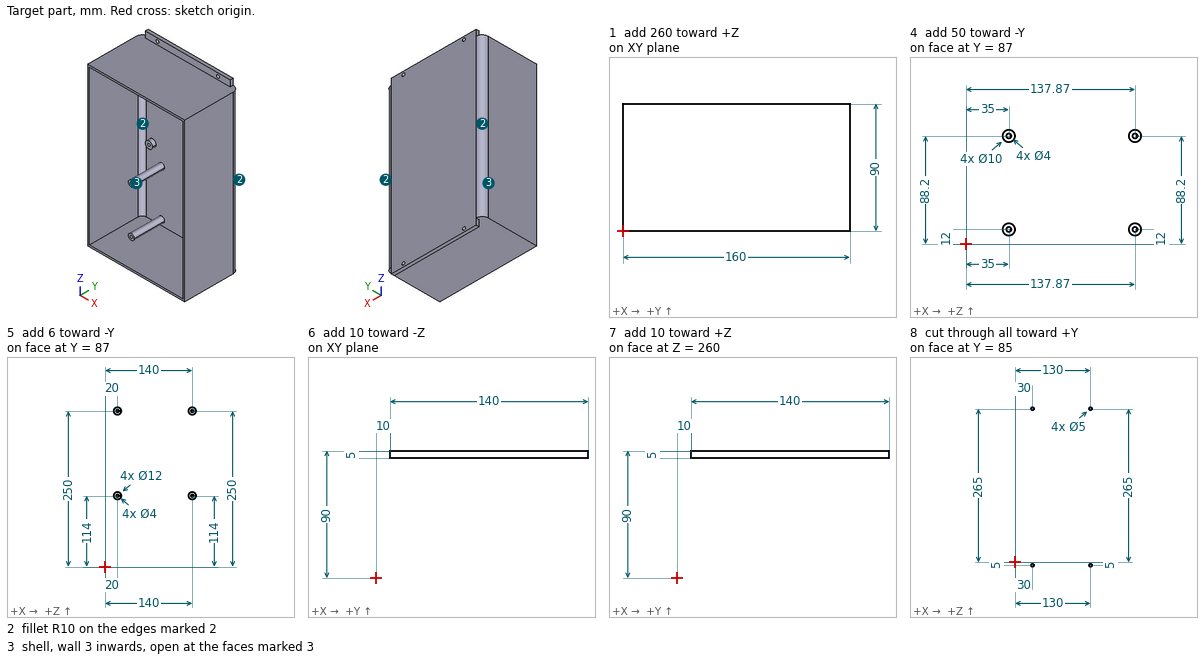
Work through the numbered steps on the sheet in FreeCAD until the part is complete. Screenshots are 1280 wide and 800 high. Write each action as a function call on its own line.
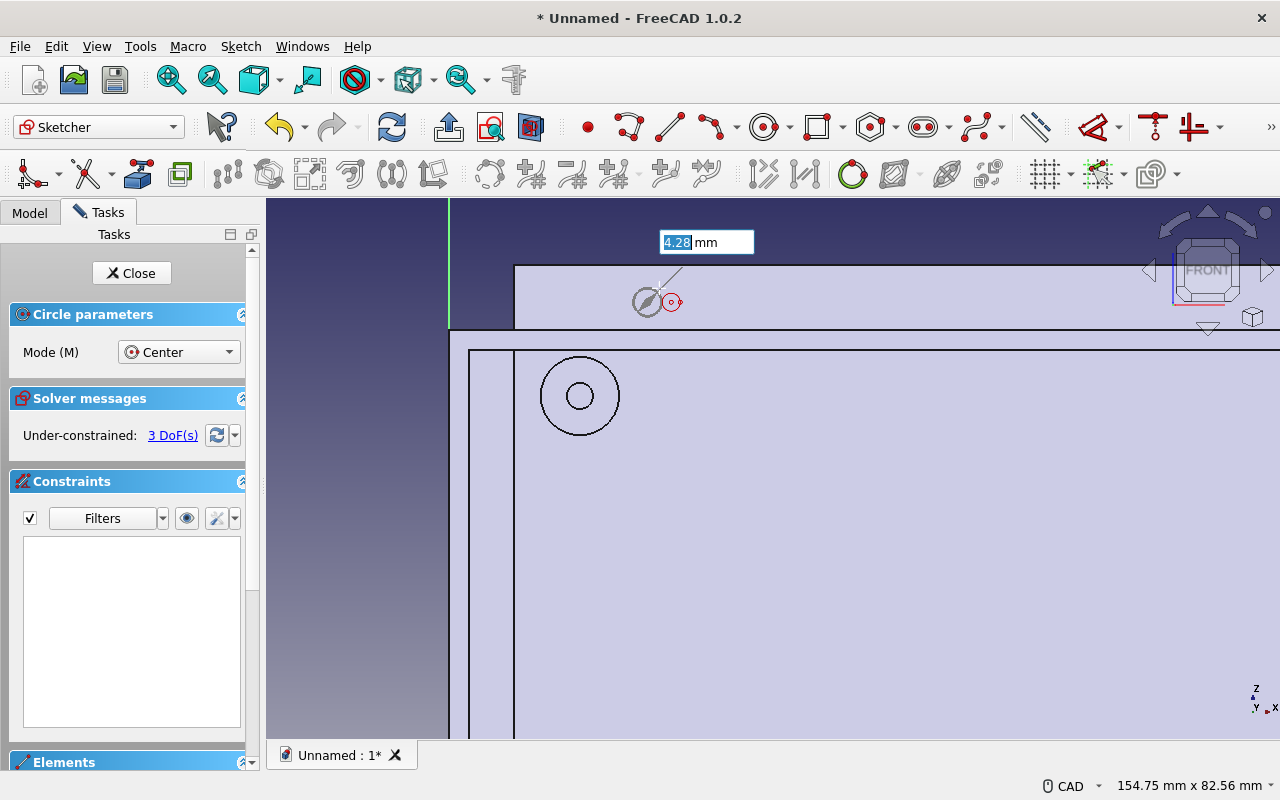
click(657, 286)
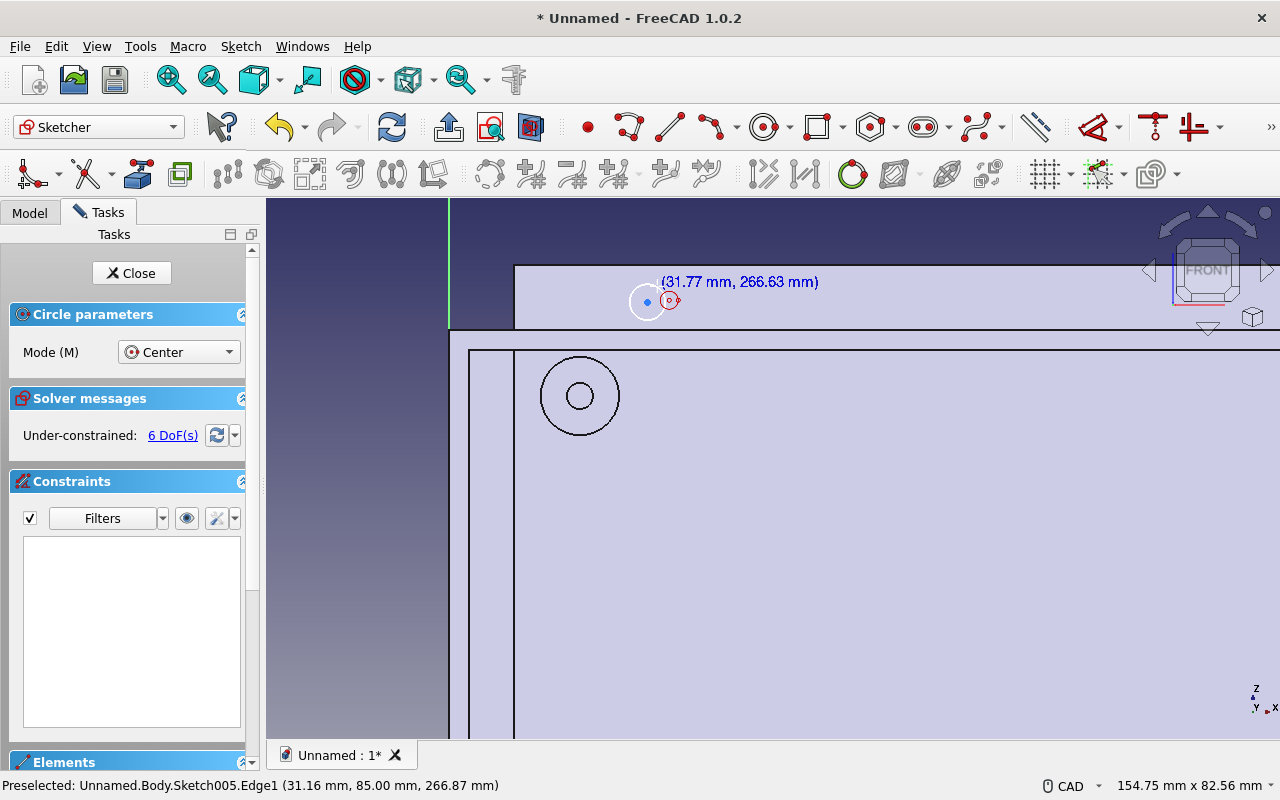
scroll(659, 288, down, 8)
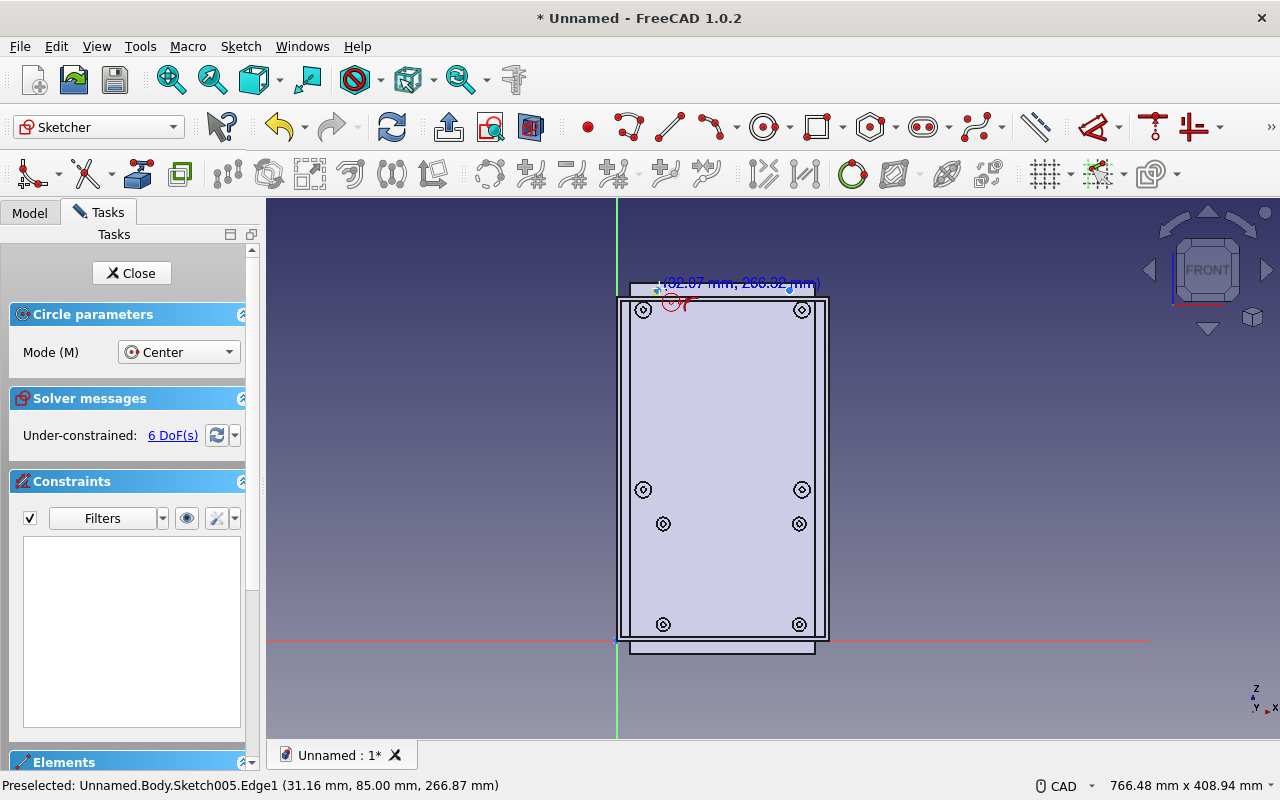
scroll(789, 647, up, 10)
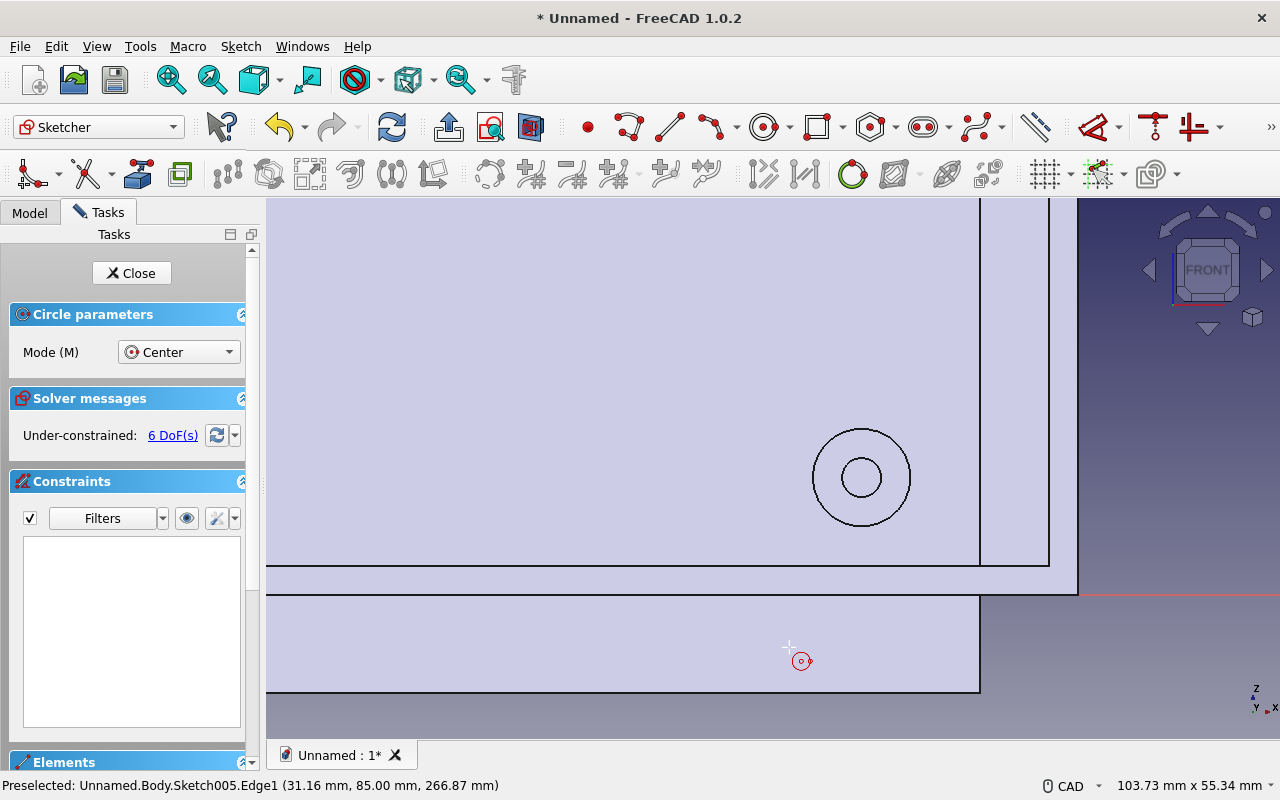
scroll(789, 648, down, 10)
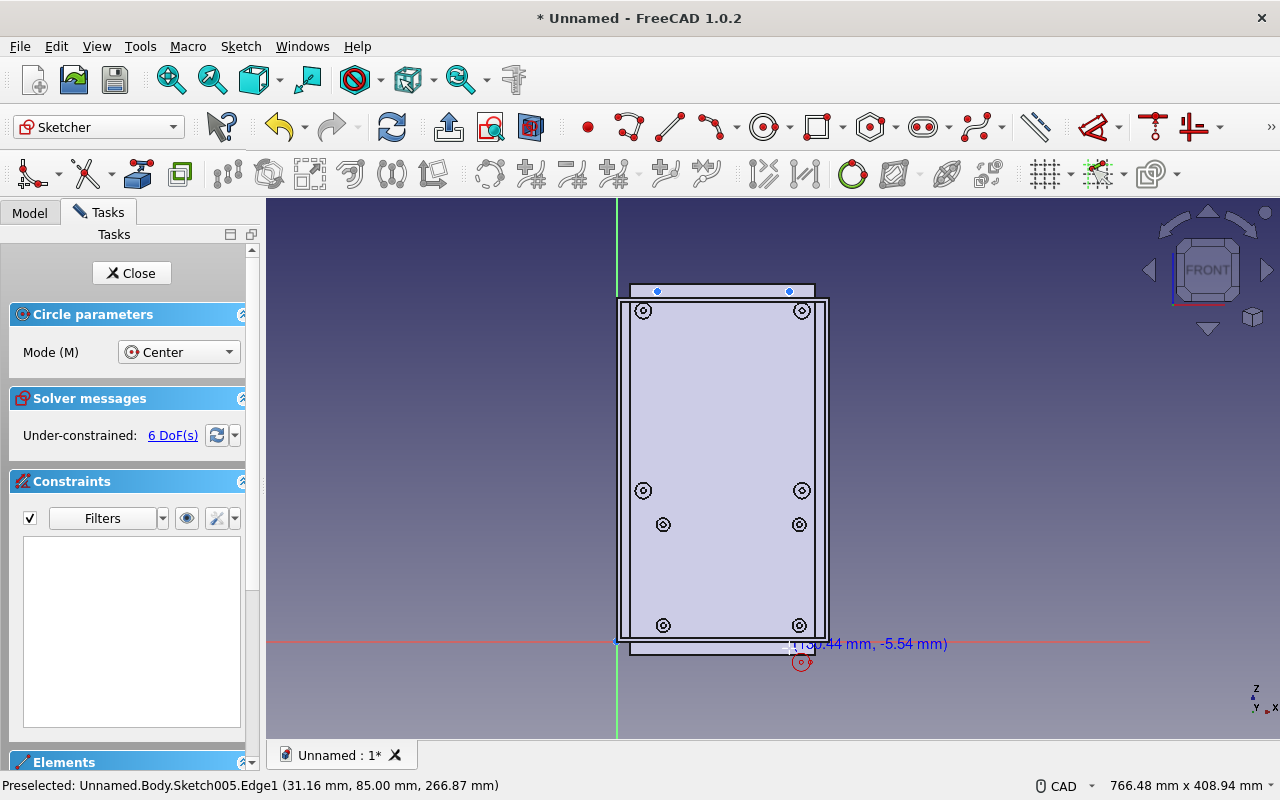
scroll(789, 648, up, 5)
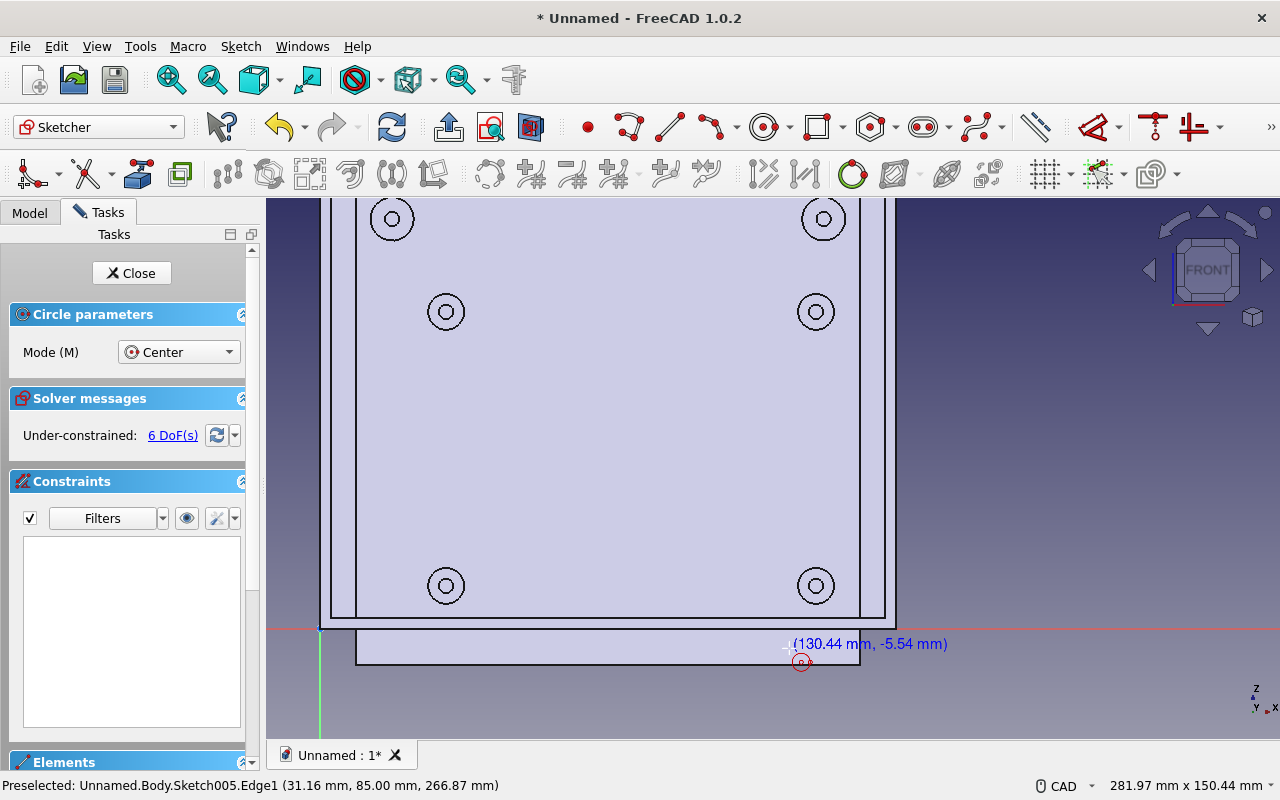
click(788, 647)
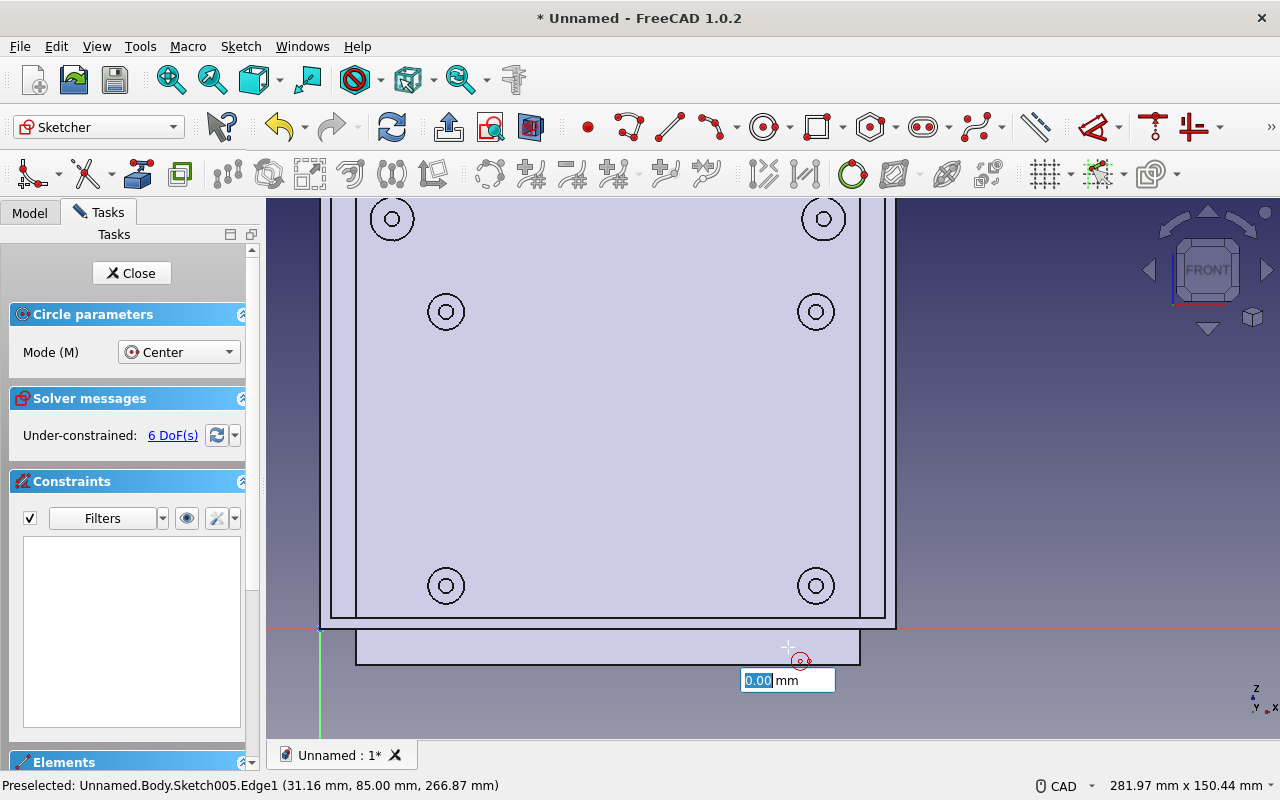
scroll(794, 653, up, 3)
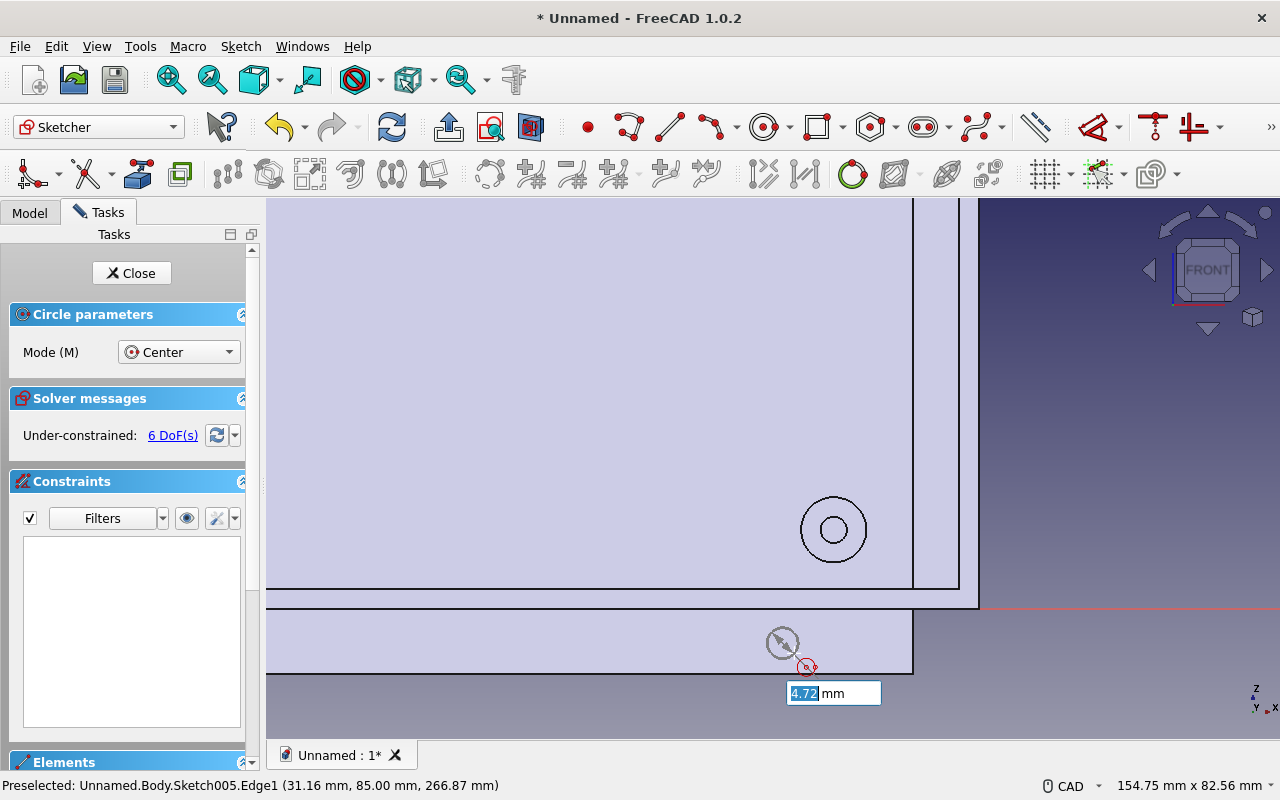
click(794, 653)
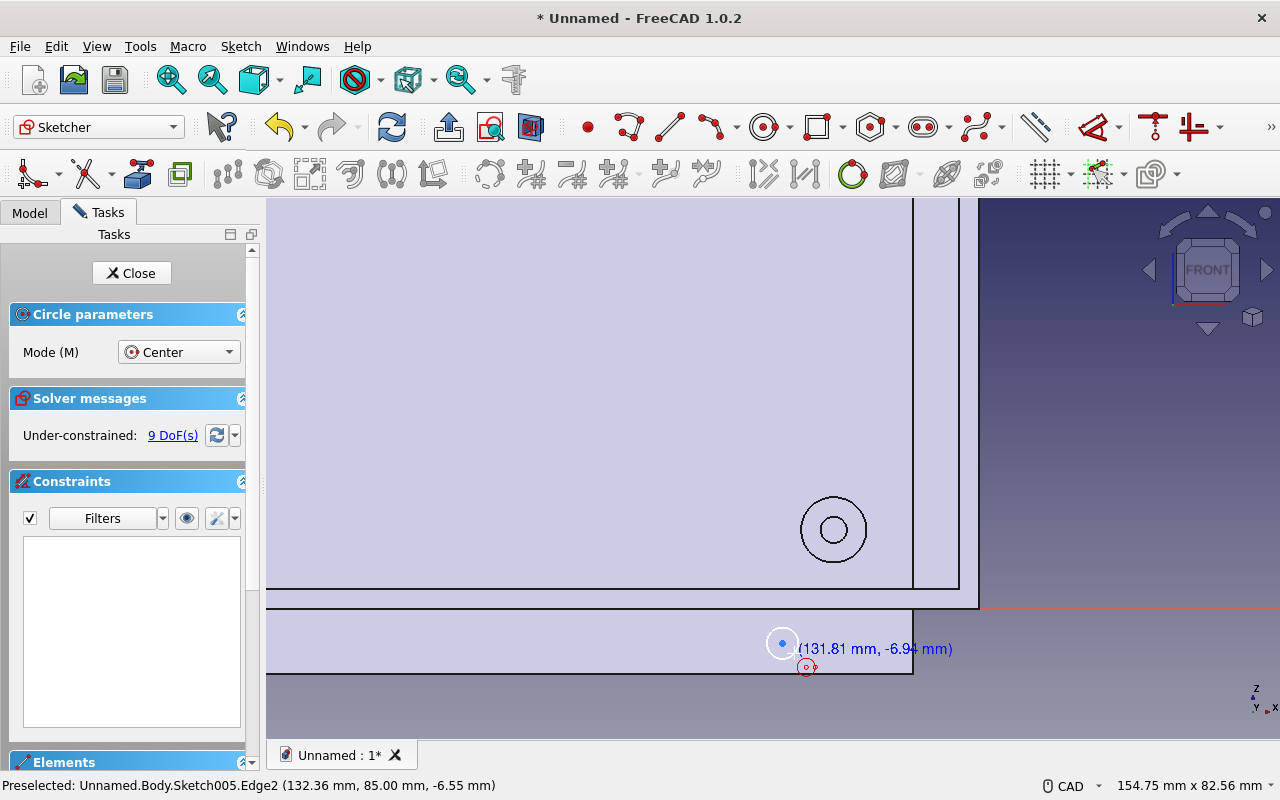
scroll(791, 649, down, 8)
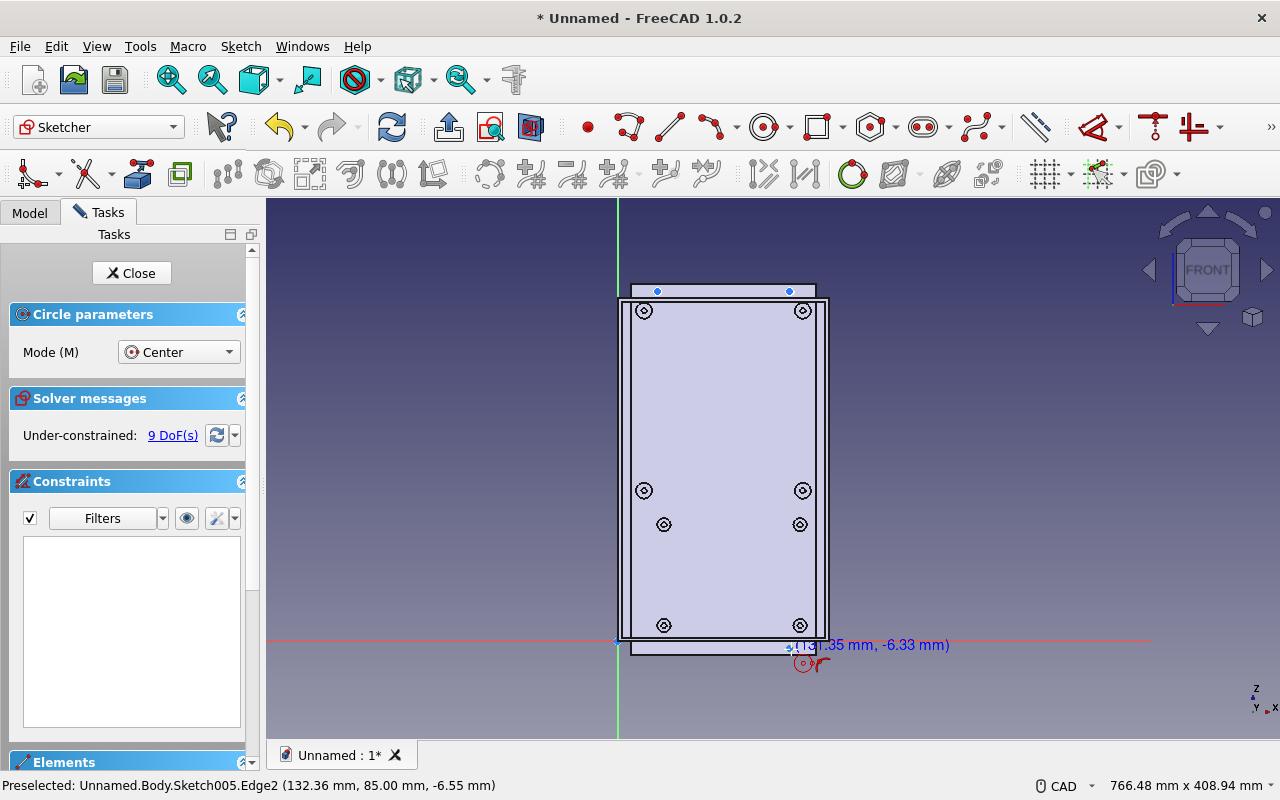
scroll(657, 648, up, 10)